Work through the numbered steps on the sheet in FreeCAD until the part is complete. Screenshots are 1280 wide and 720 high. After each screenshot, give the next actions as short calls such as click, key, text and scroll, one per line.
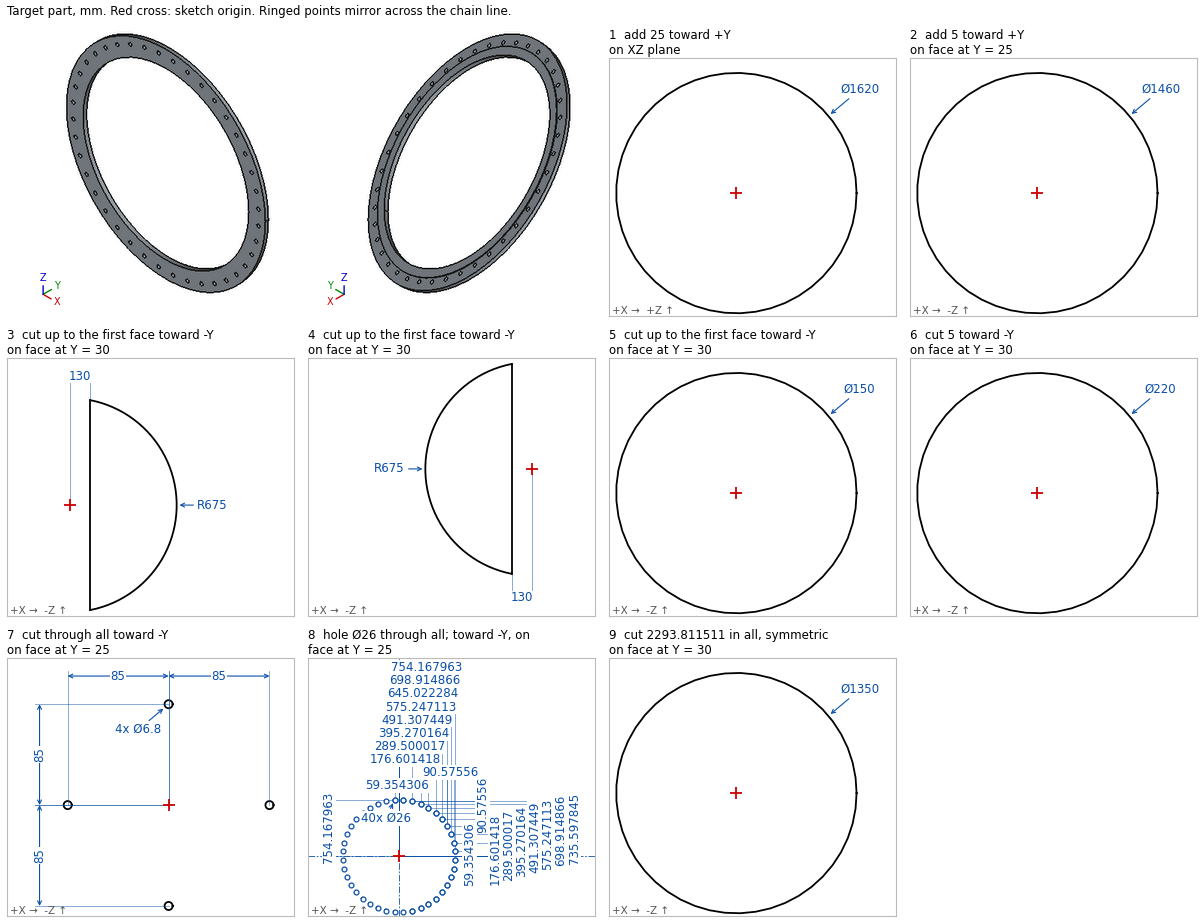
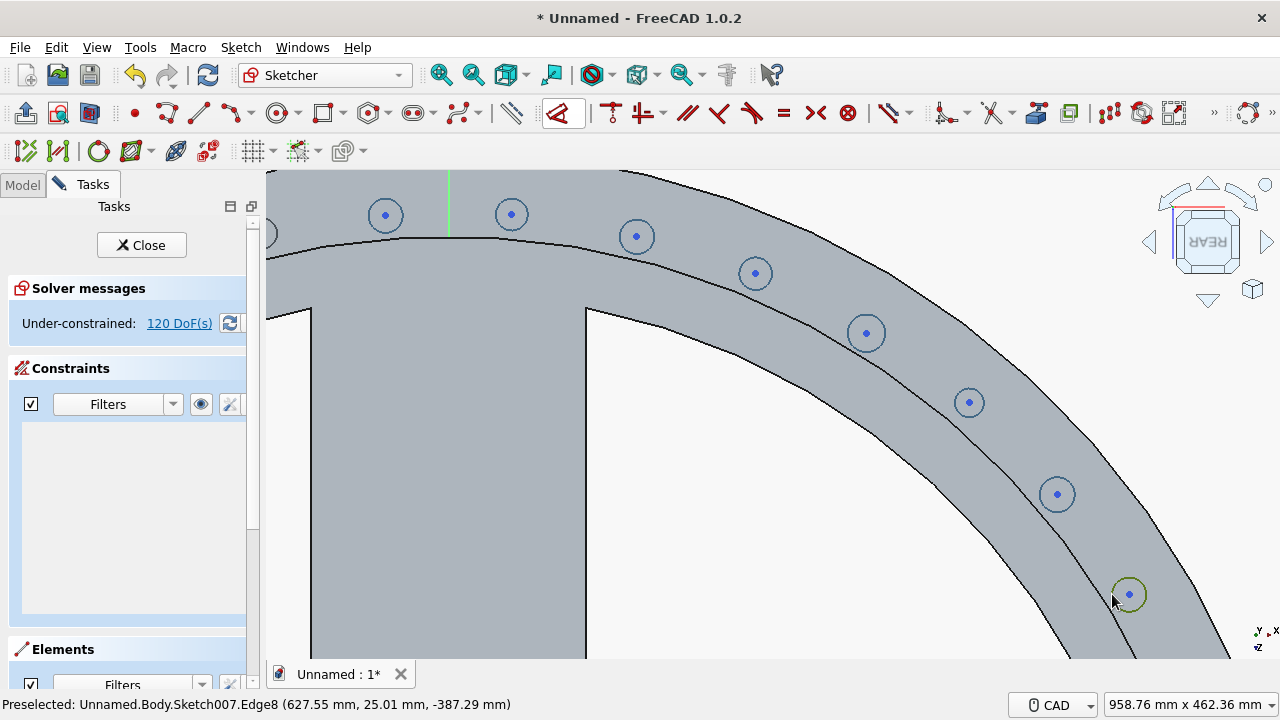
scroll(769, 264, down, 8)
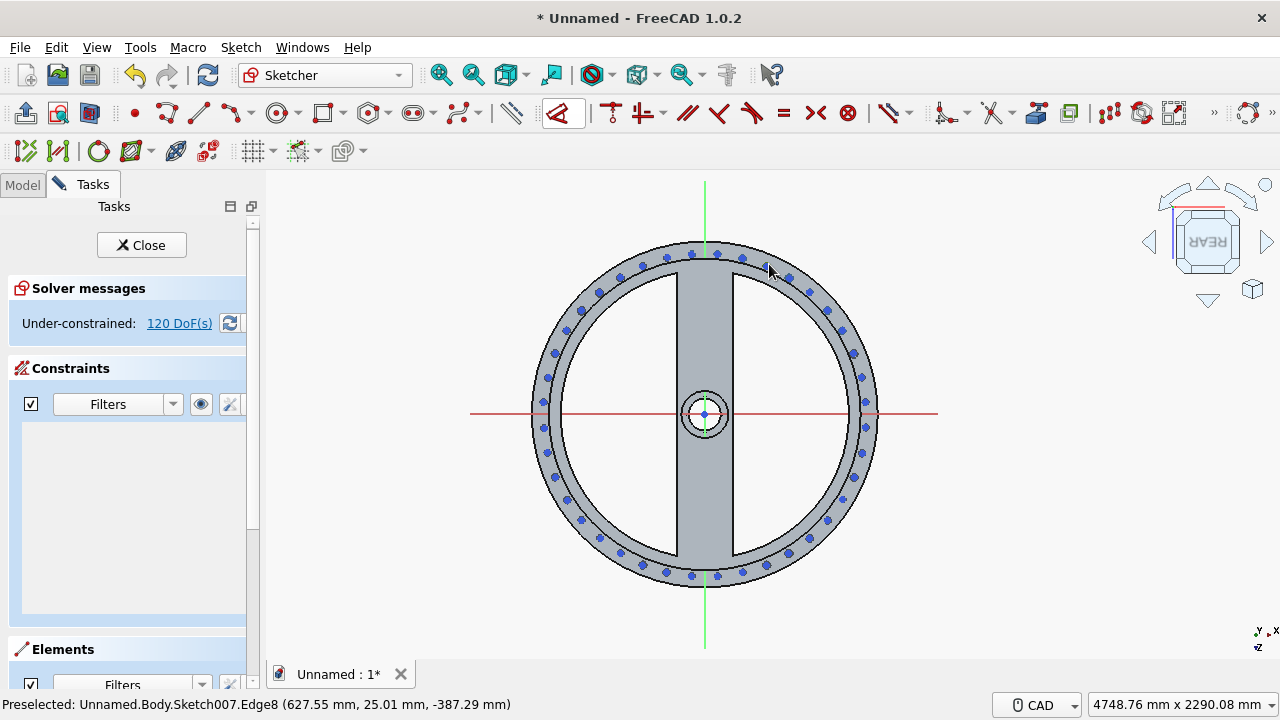
scroll(856, 351, up, 7)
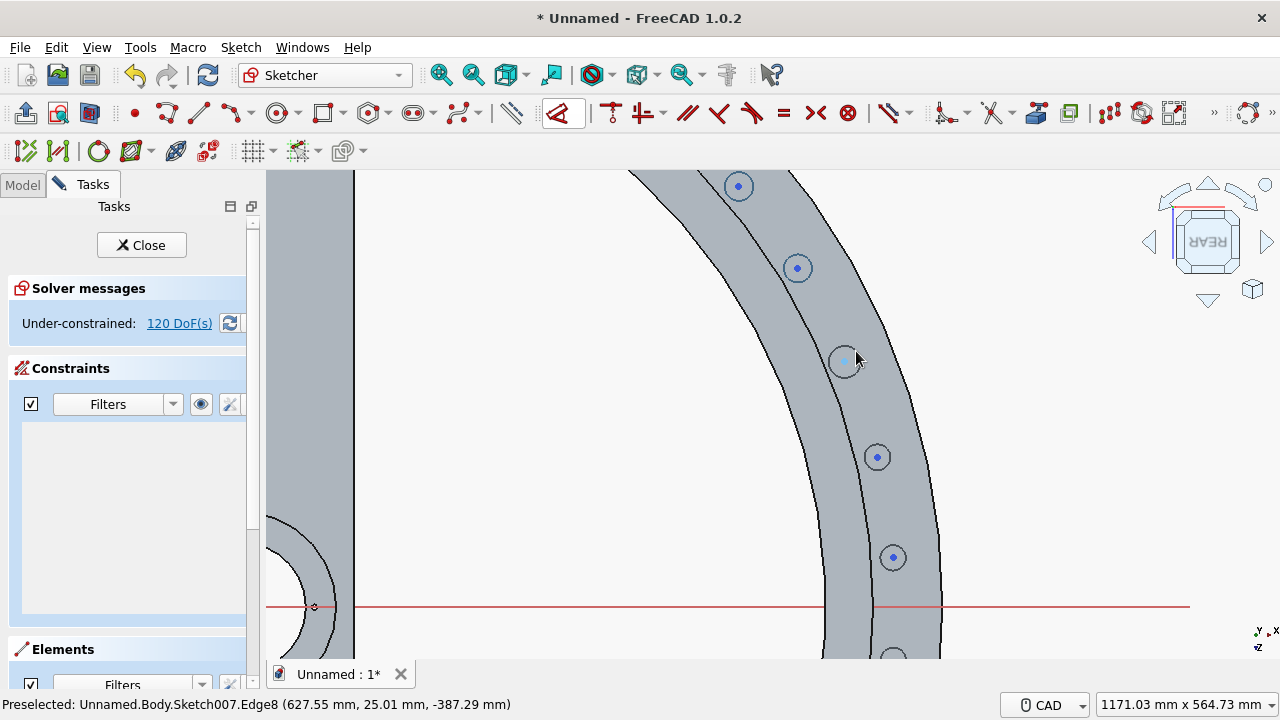
click(856, 351)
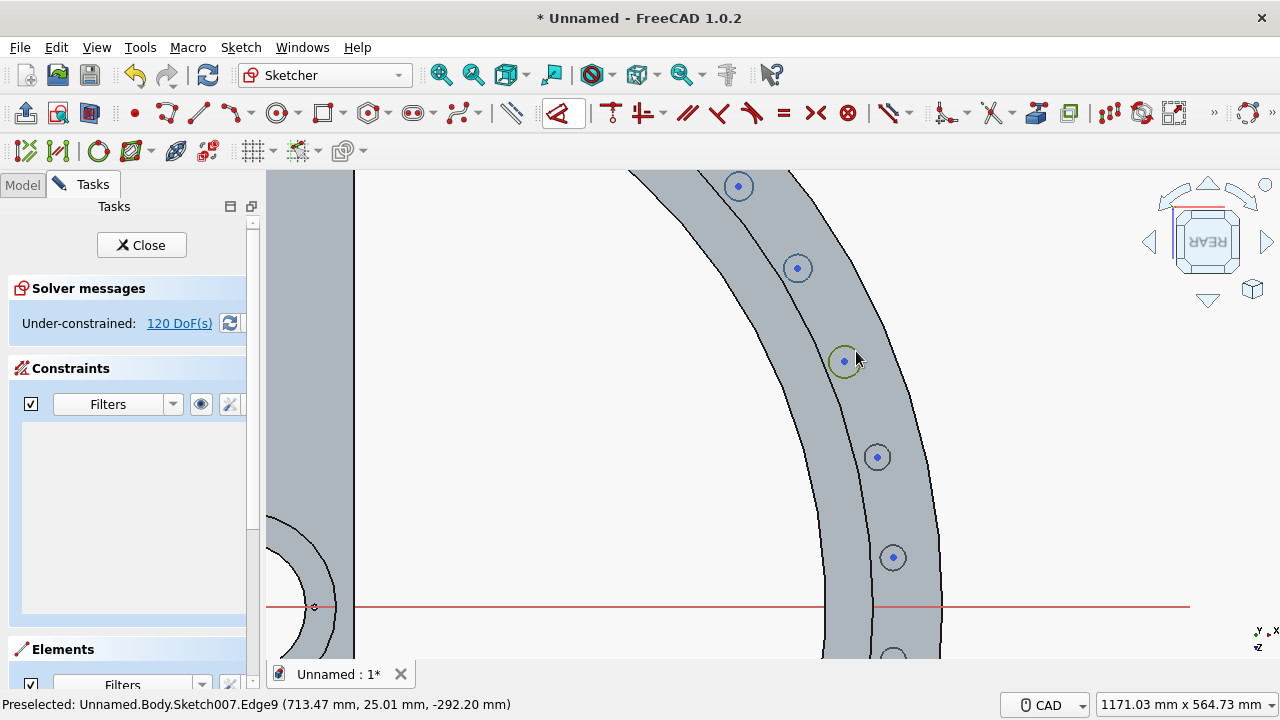
click(887, 448)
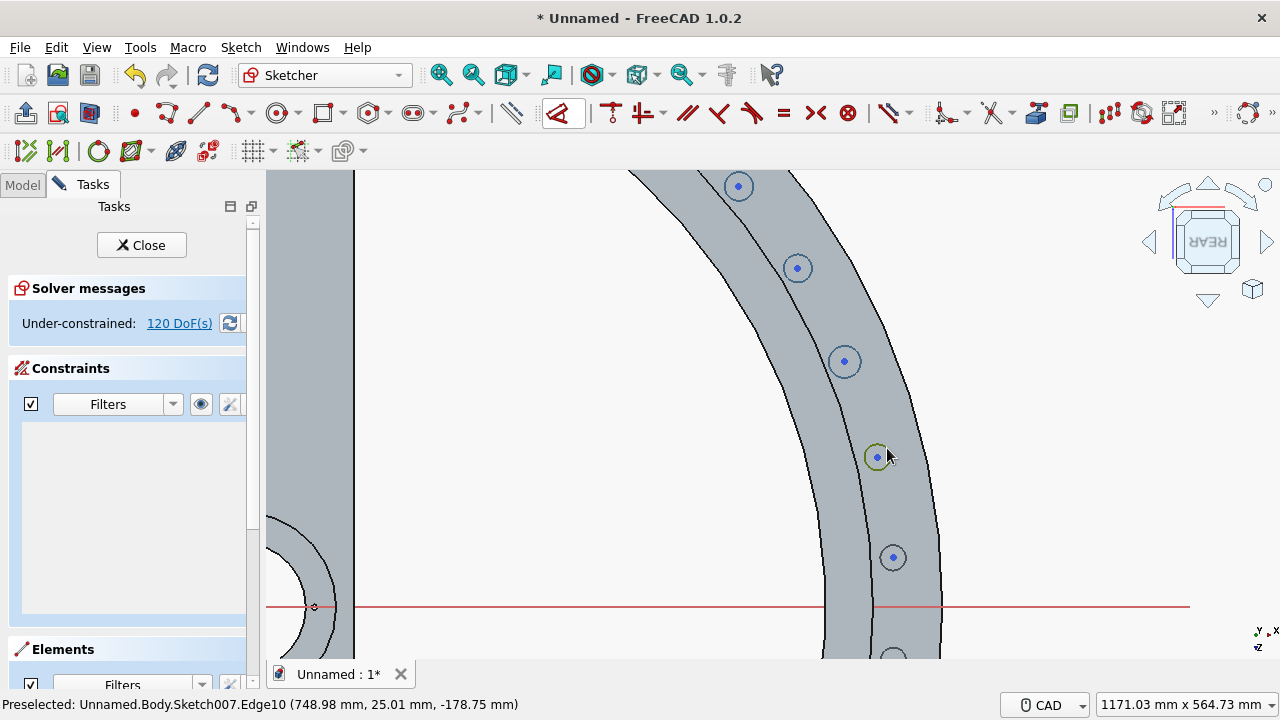
click(902, 549)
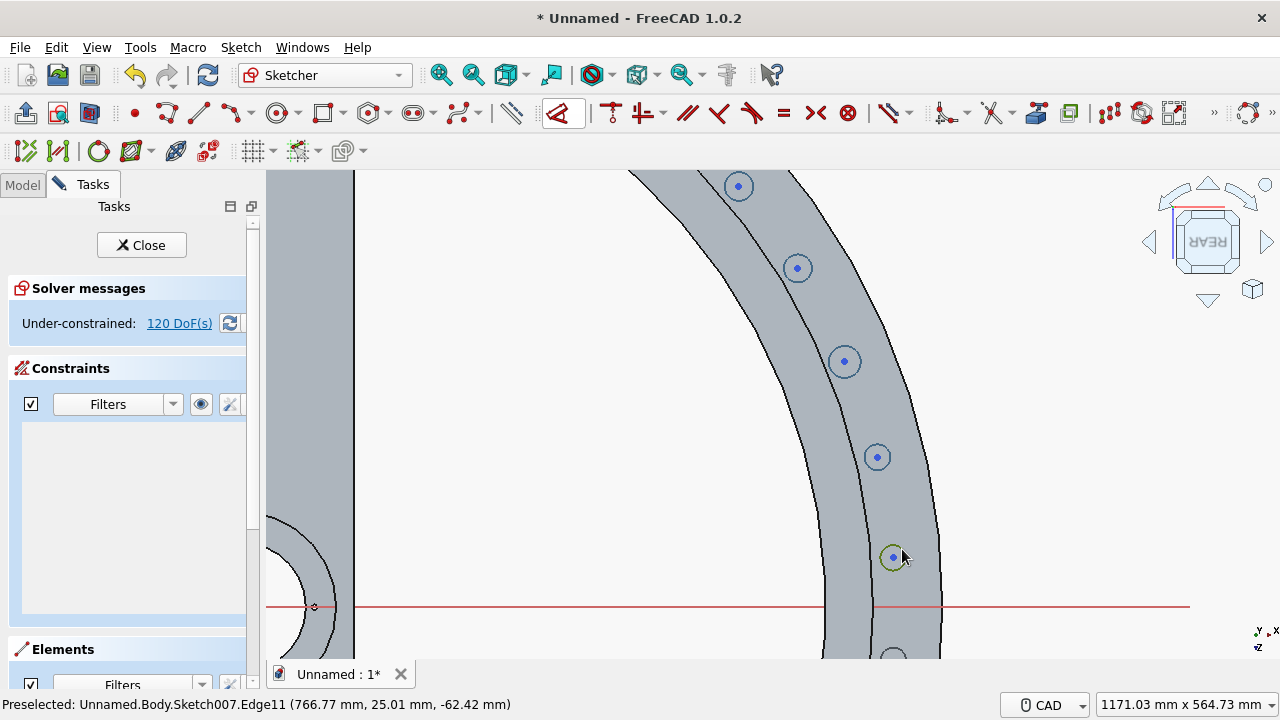
scroll(856, 351, down, 7)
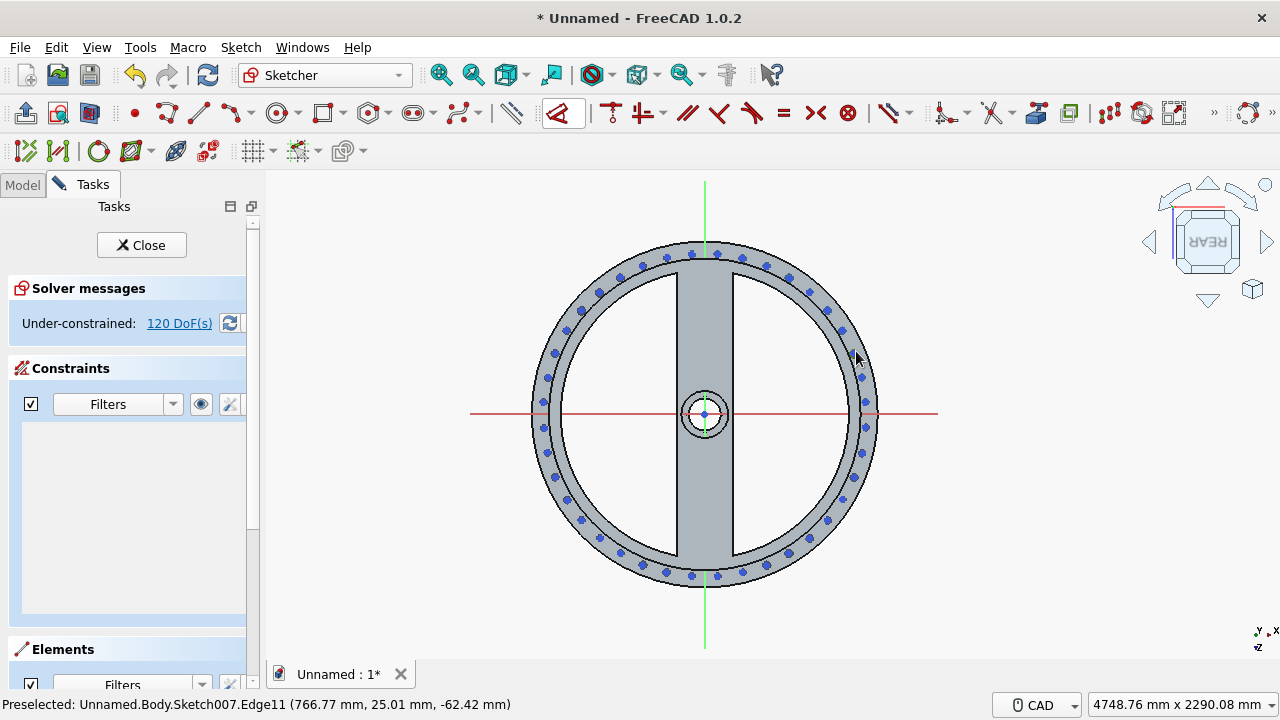
scroll(868, 425, up, 8)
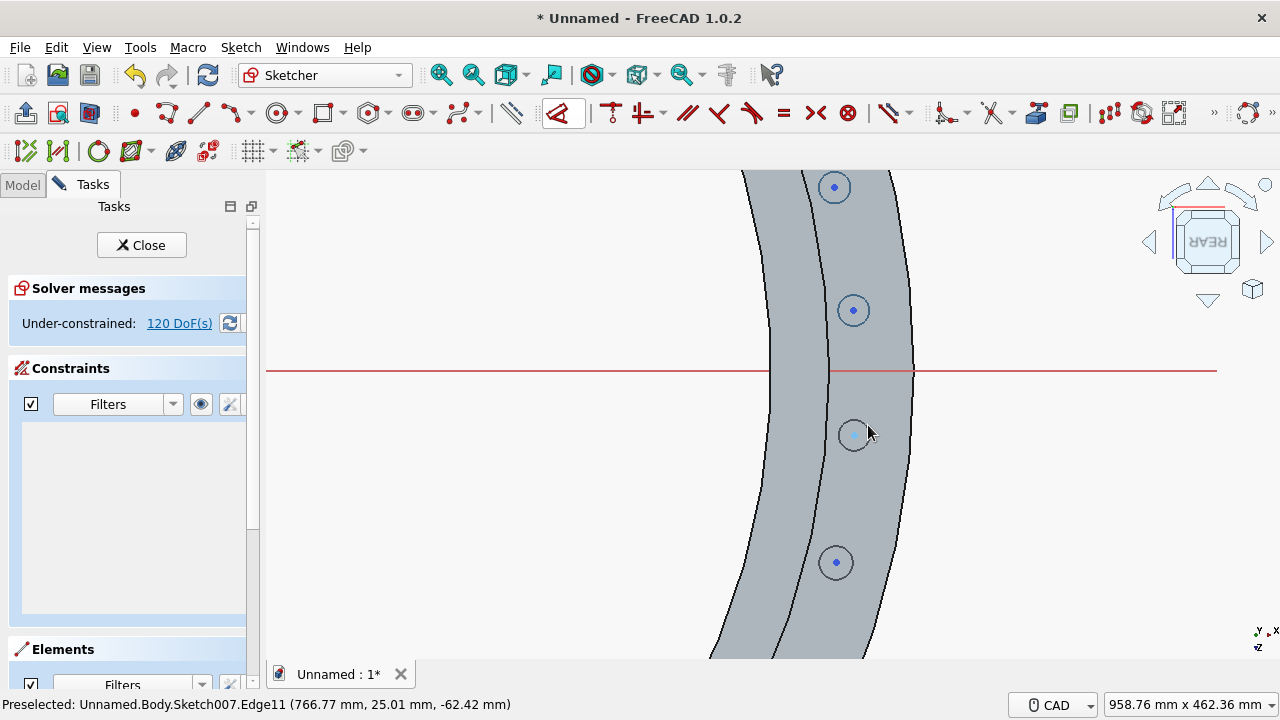
click(865, 424)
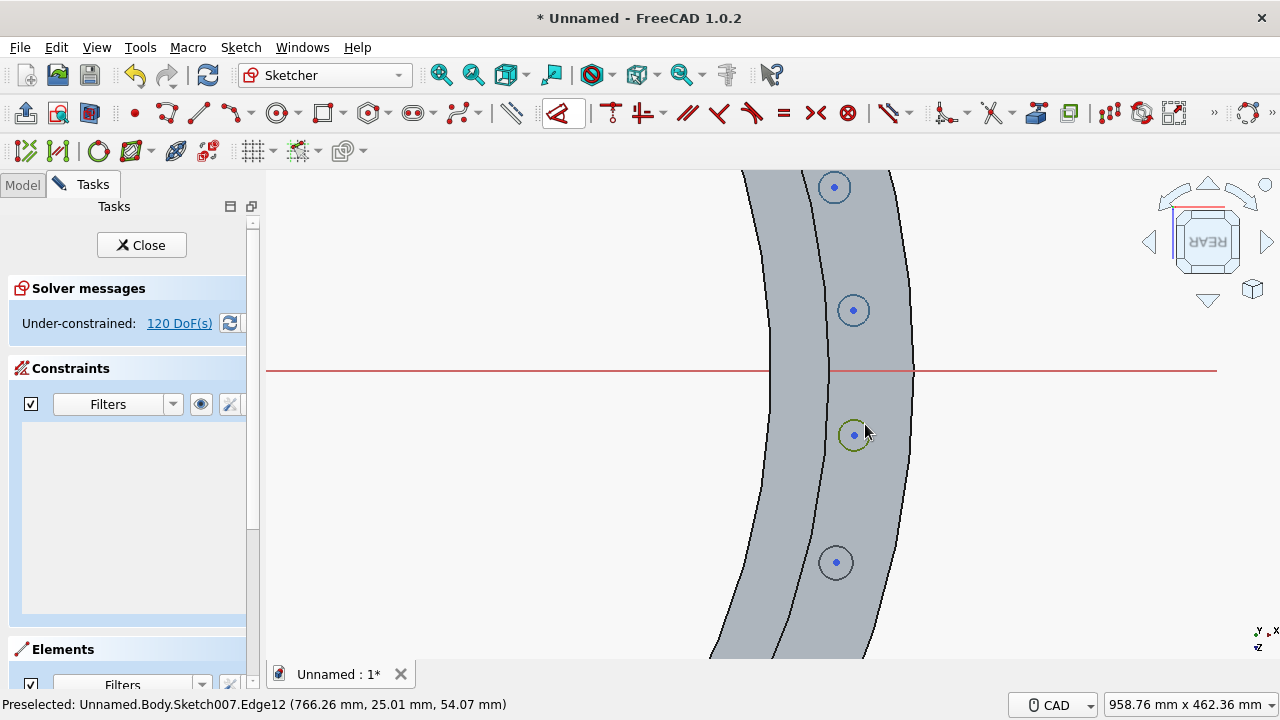
click(848, 551)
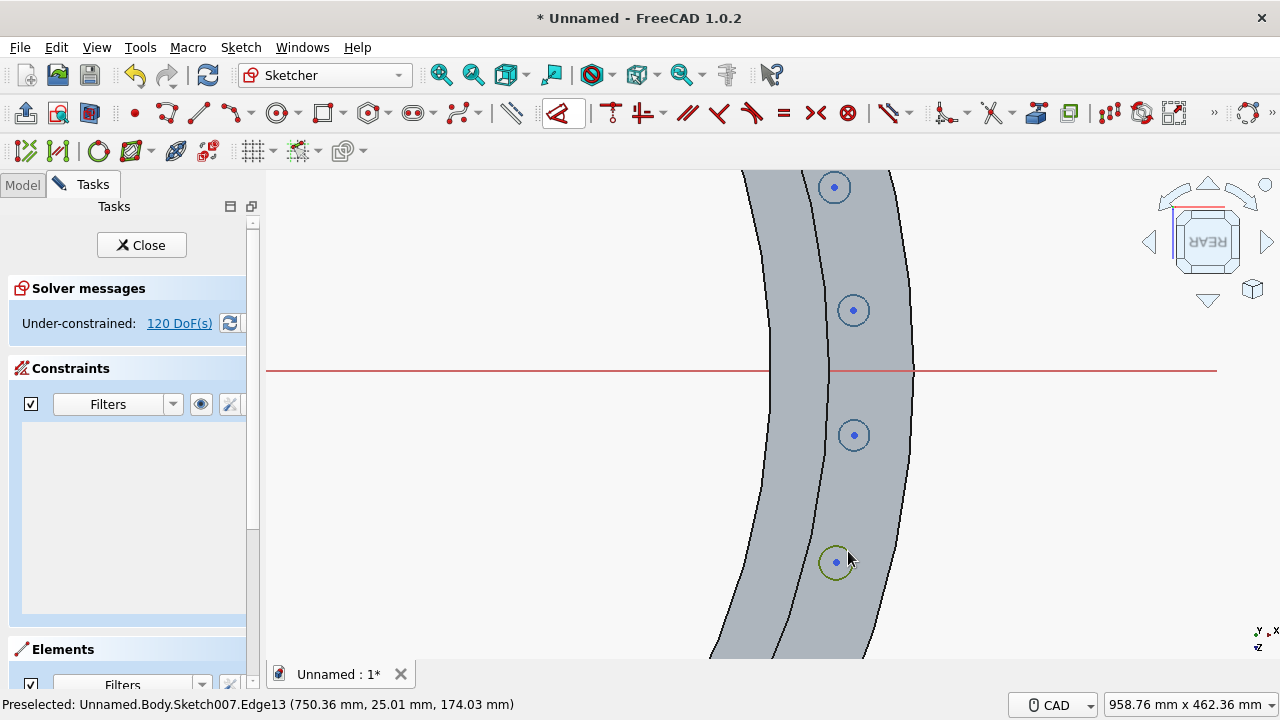
scroll(868, 426, down, 8)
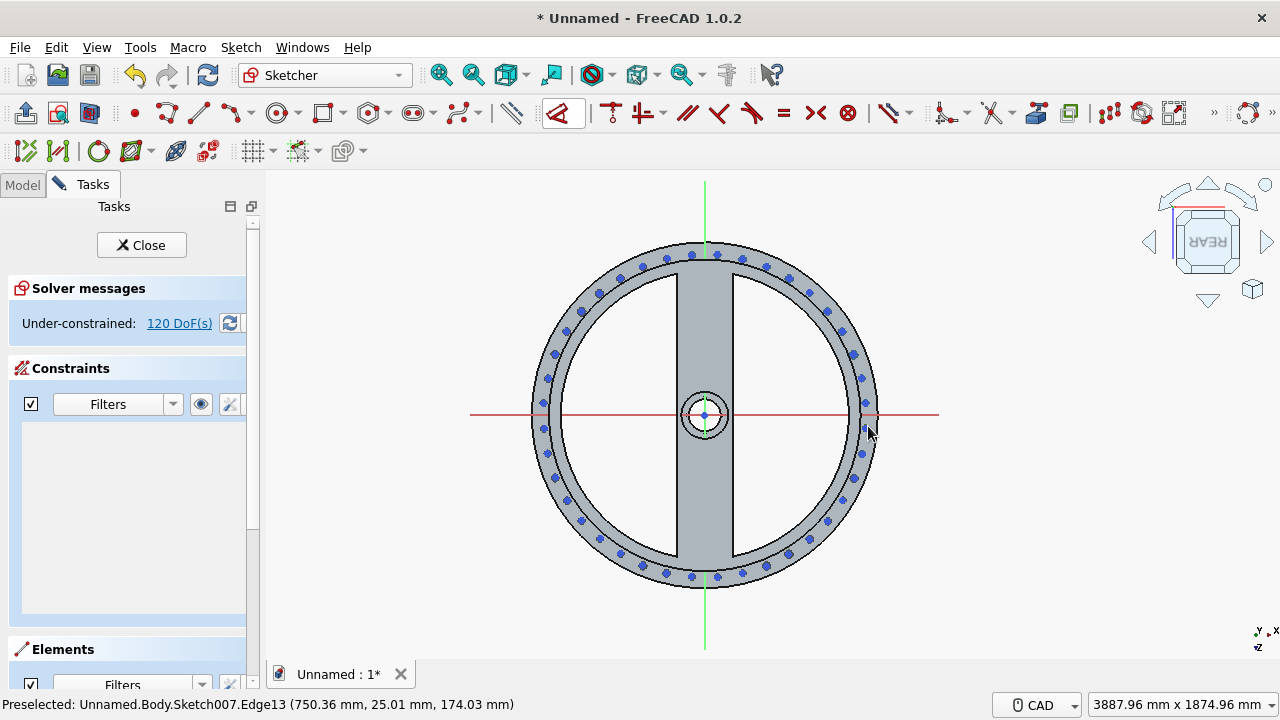
scroll(857, 476, up, 7)